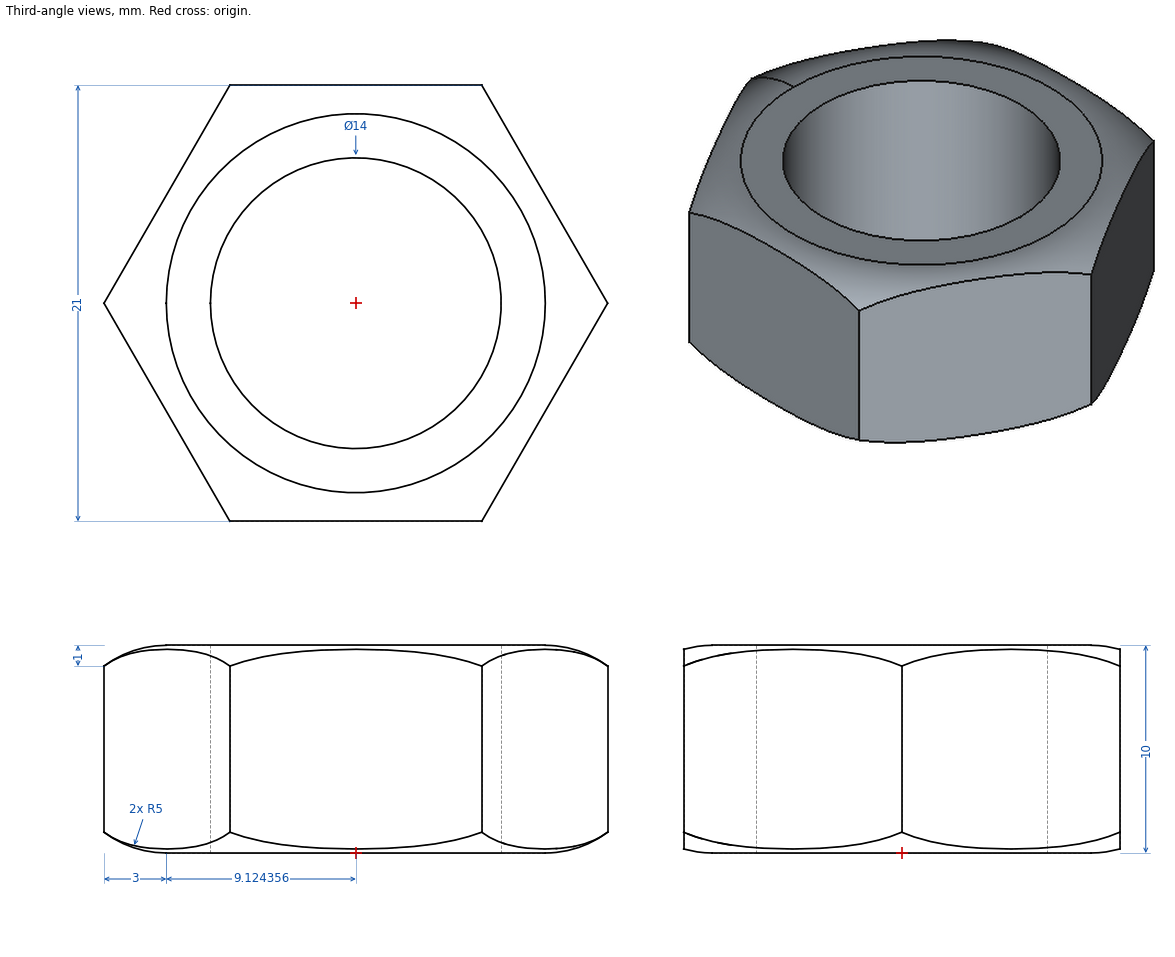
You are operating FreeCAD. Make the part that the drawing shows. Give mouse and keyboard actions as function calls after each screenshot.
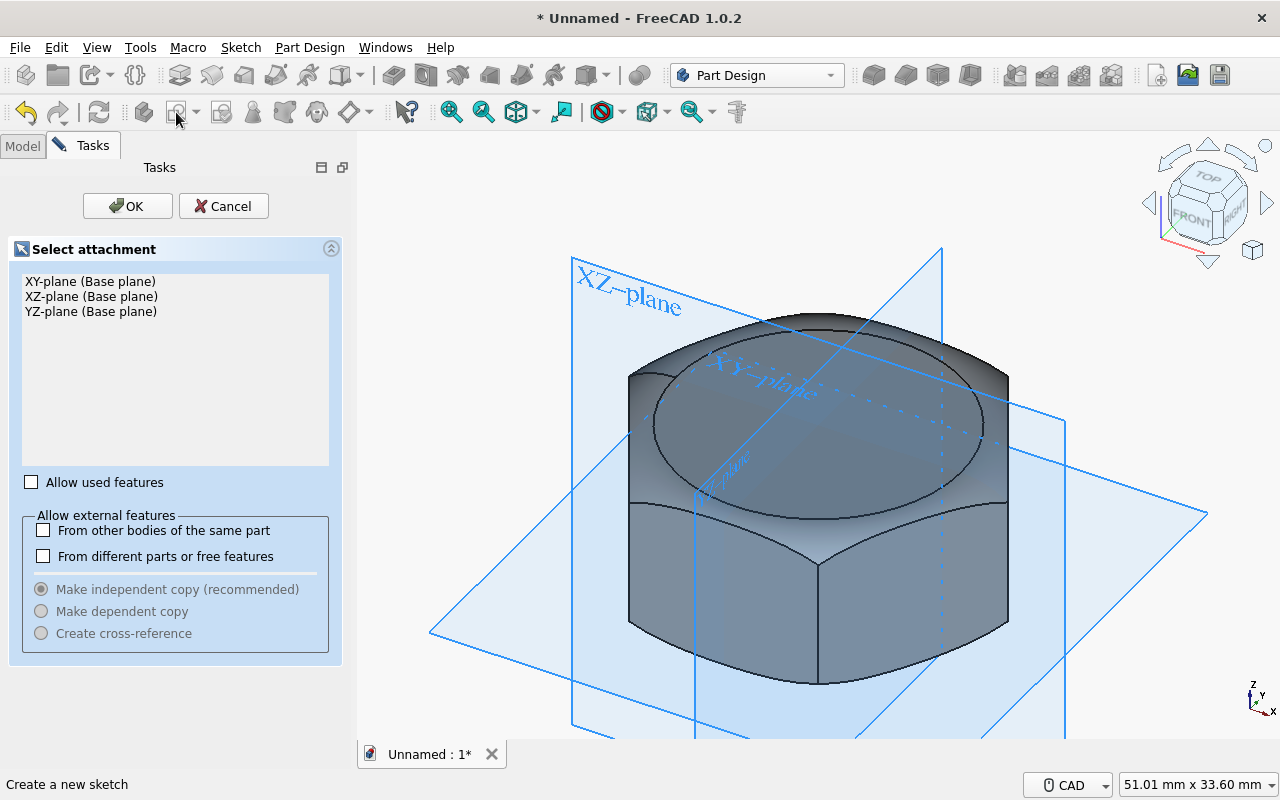
click(82, 282)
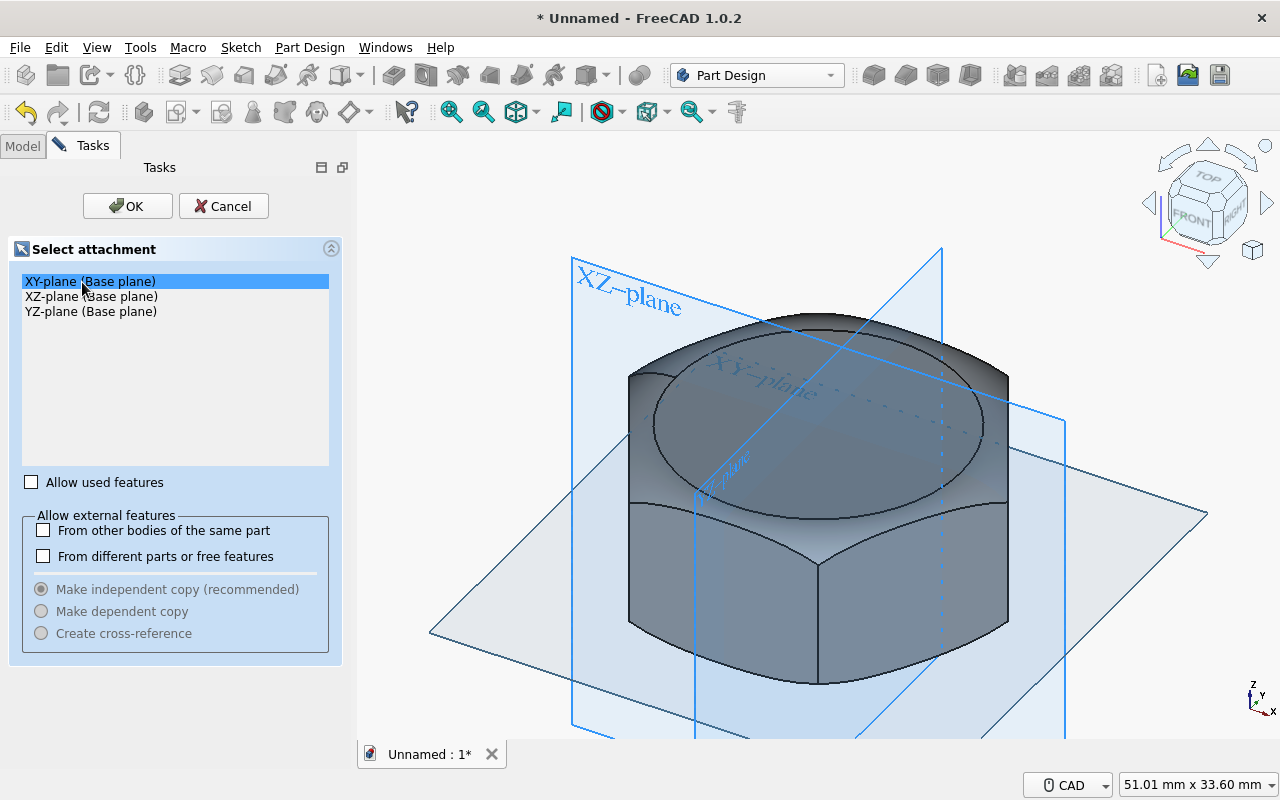
click(128, 206)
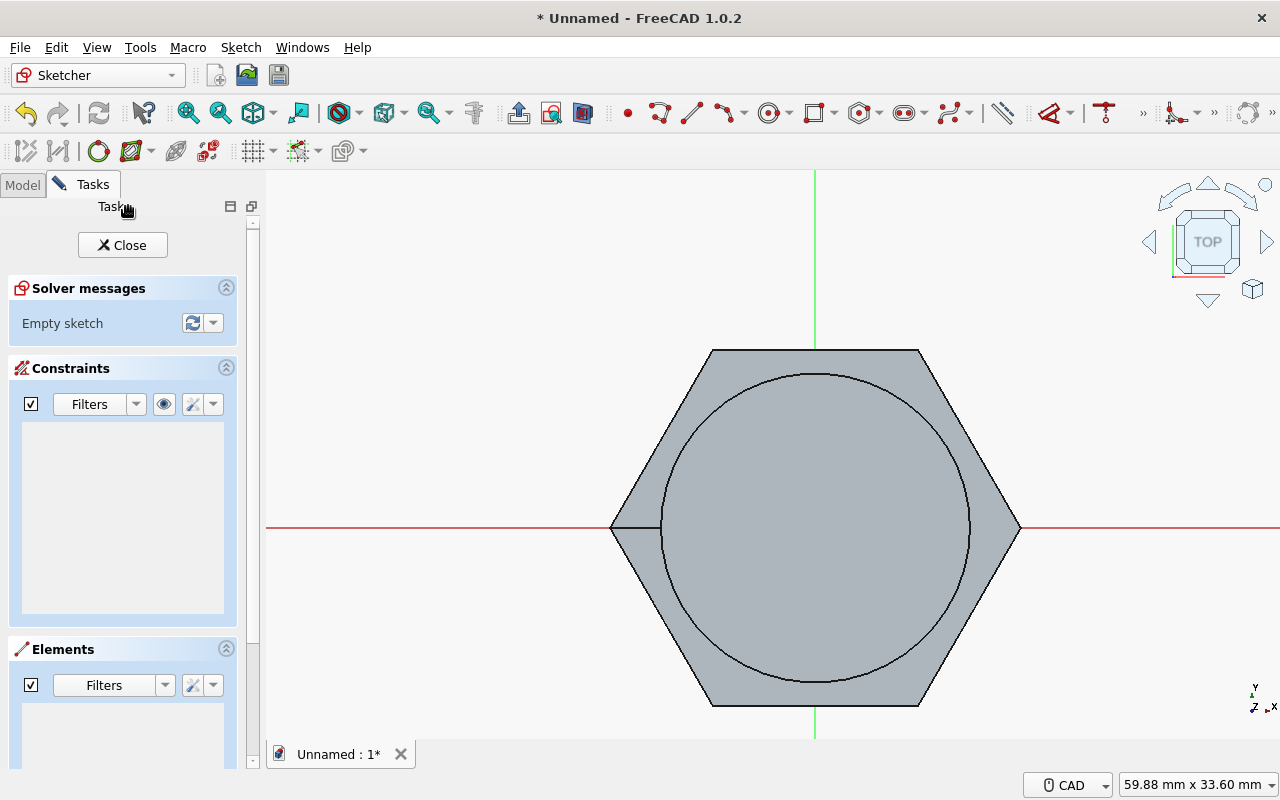
key(q)
key(s)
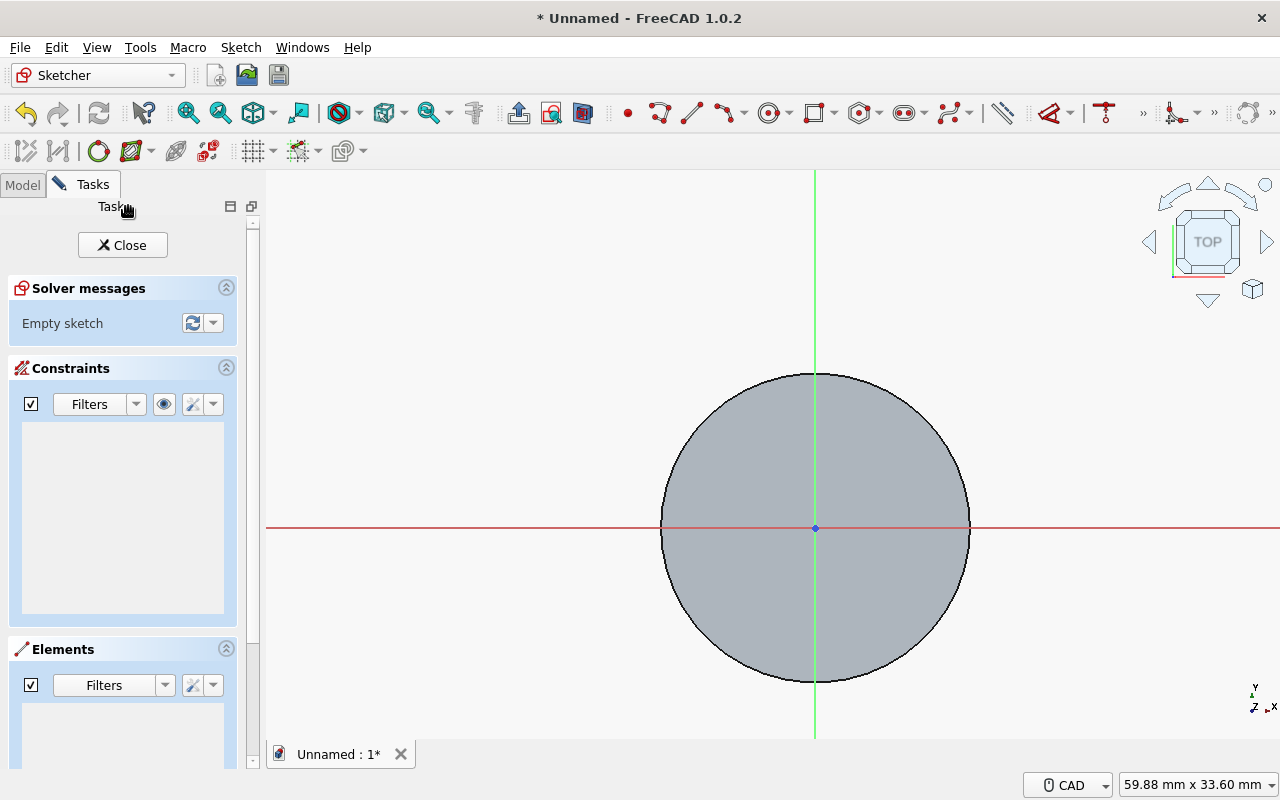
scroll(1041, 678, up, 2)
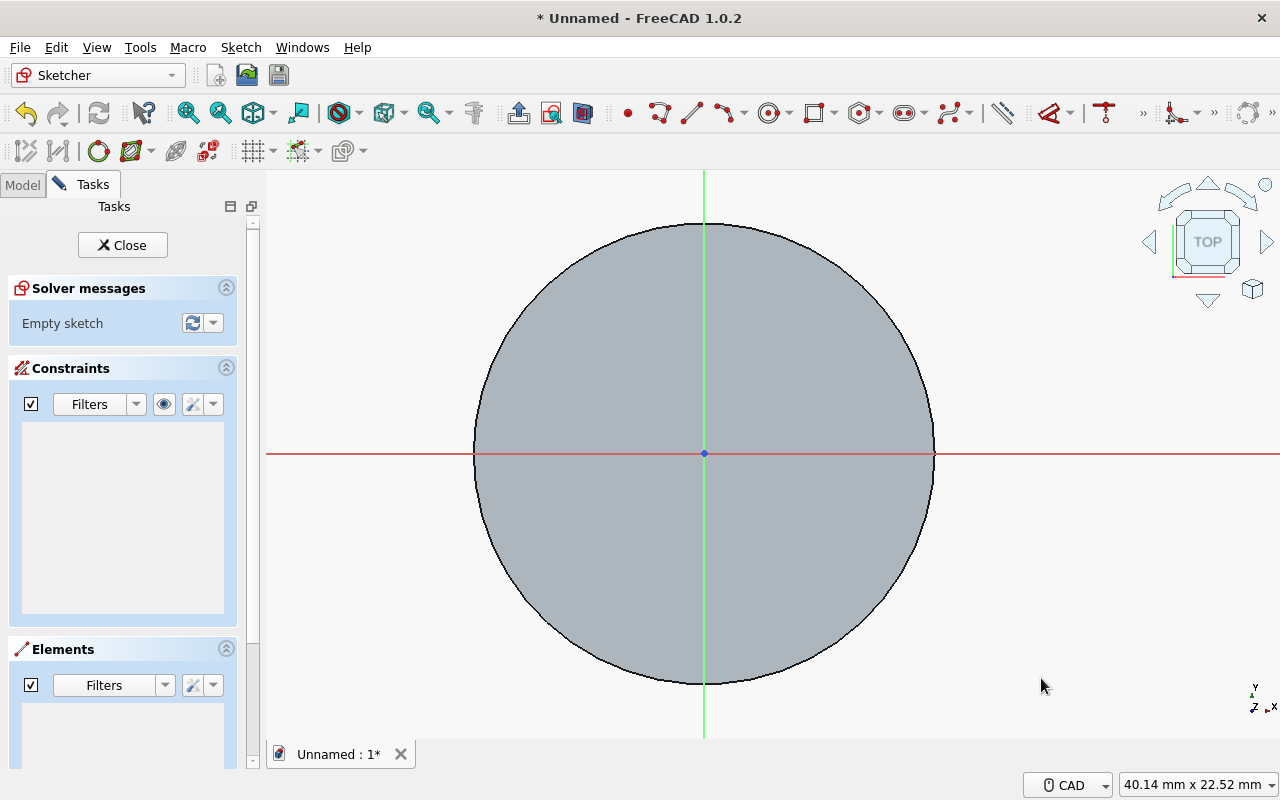
key(g)
key(c)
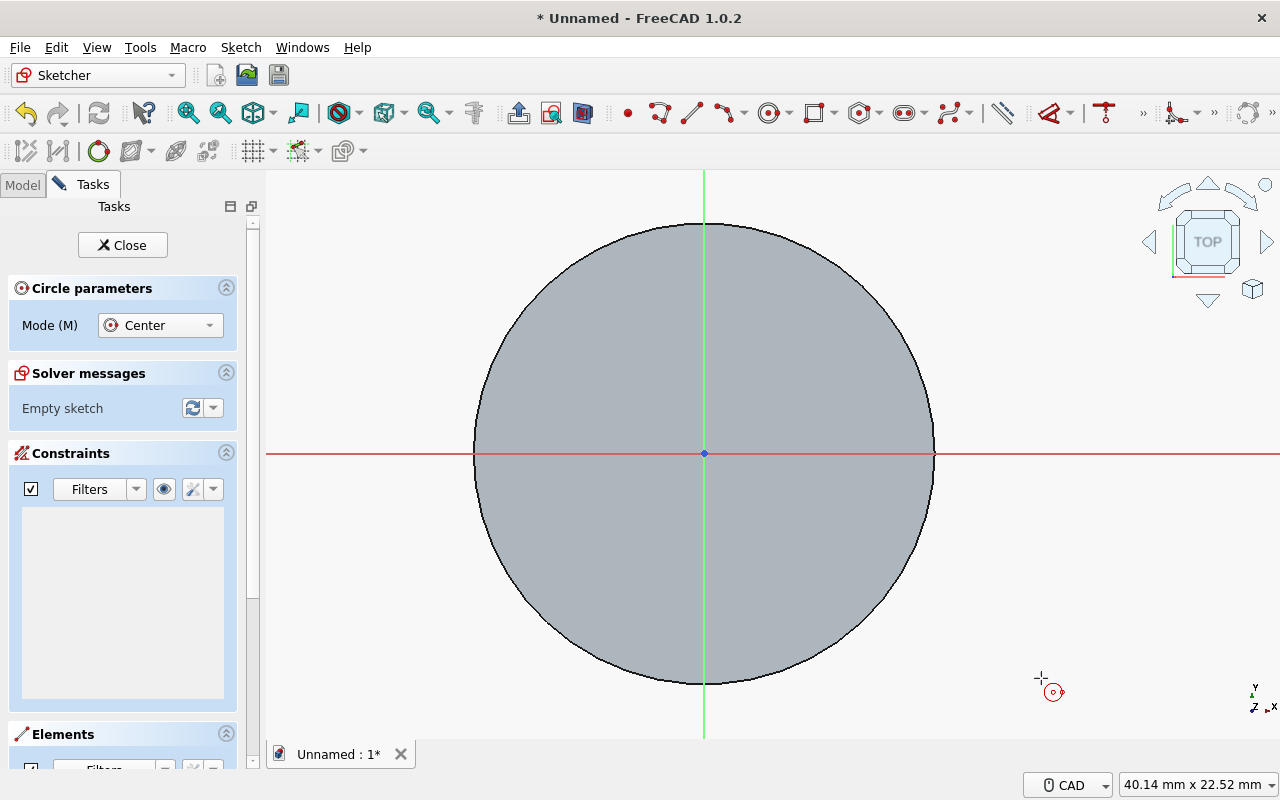
click(704, 454)
move(829, 329)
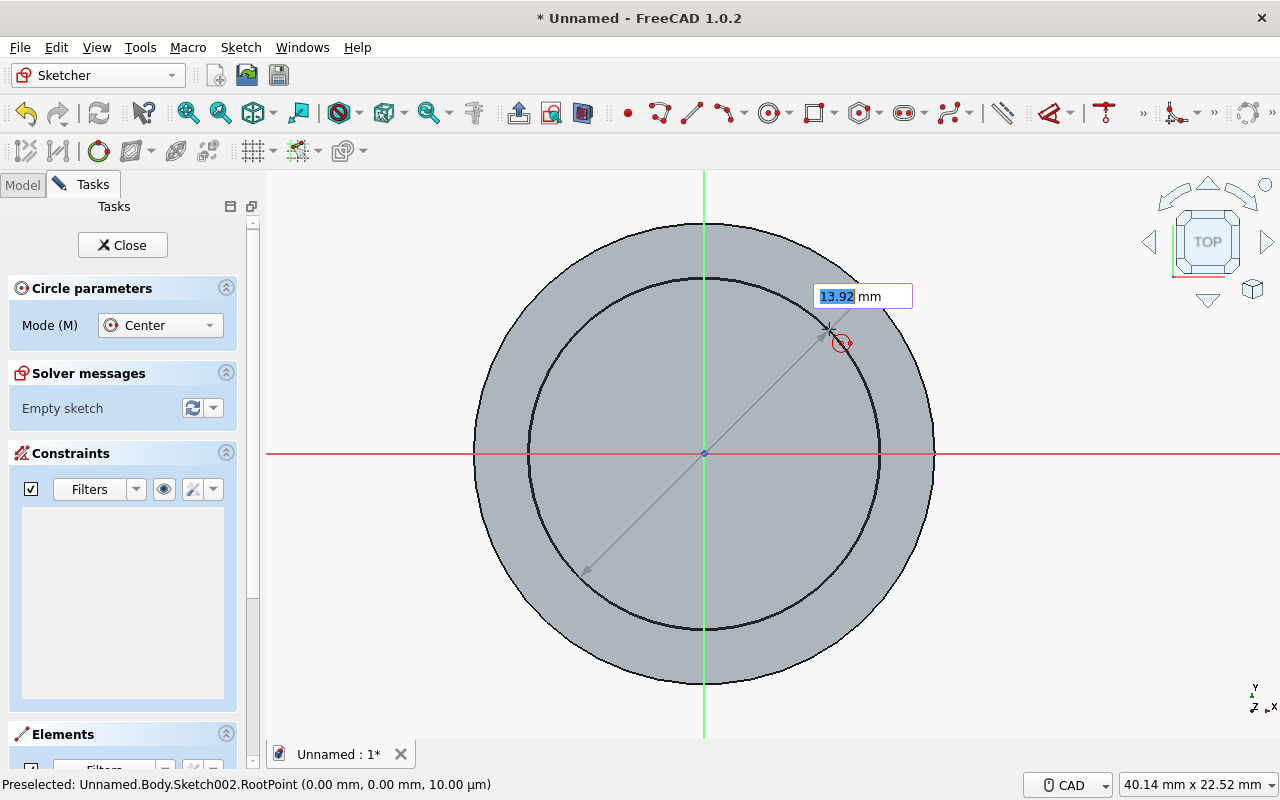
text(14)
key(Return)
key(Escape)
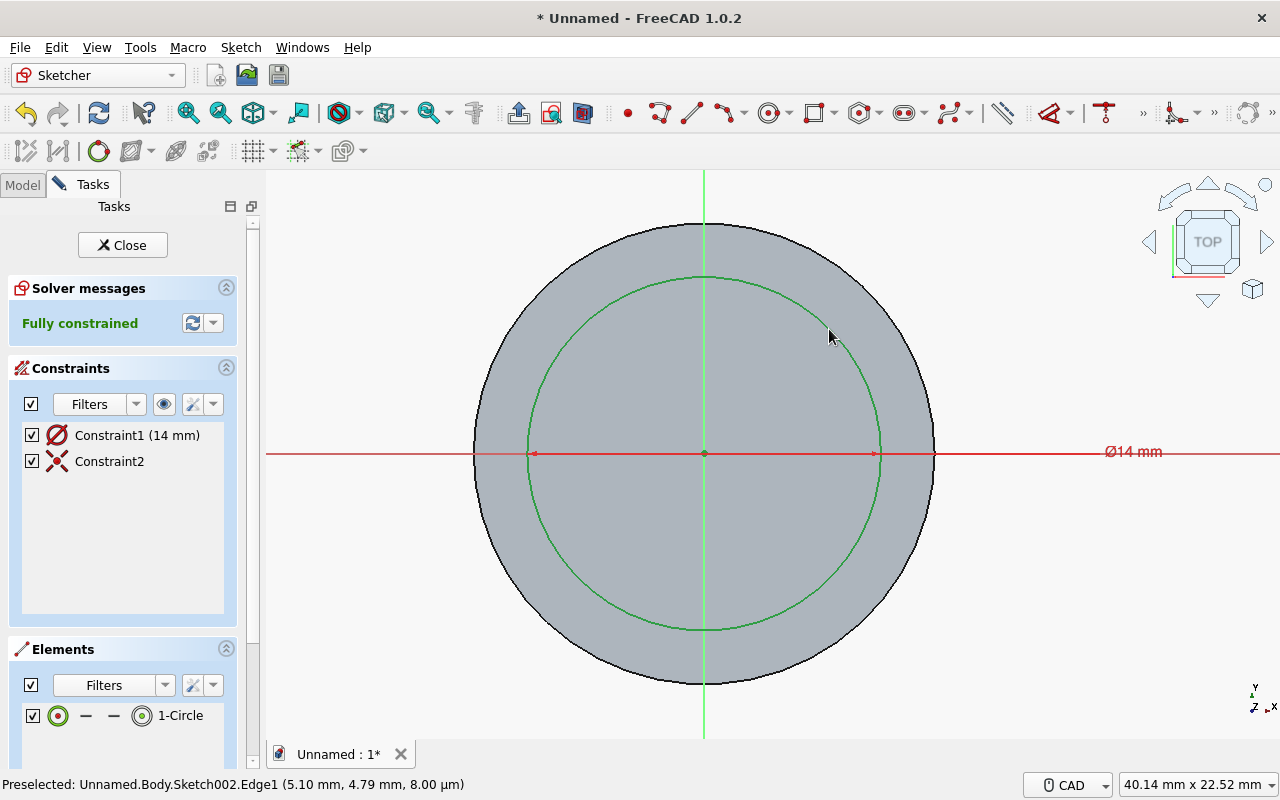
click(123, 245)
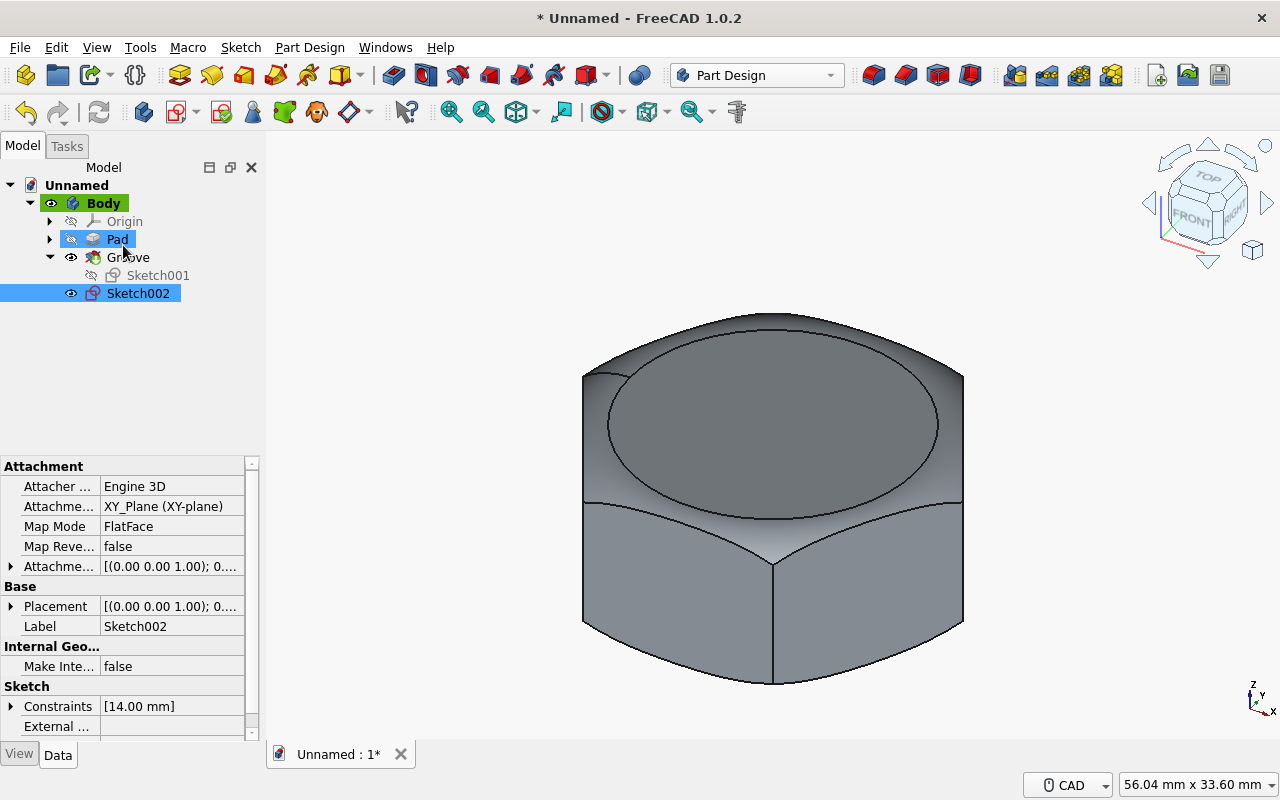
click(394, 76)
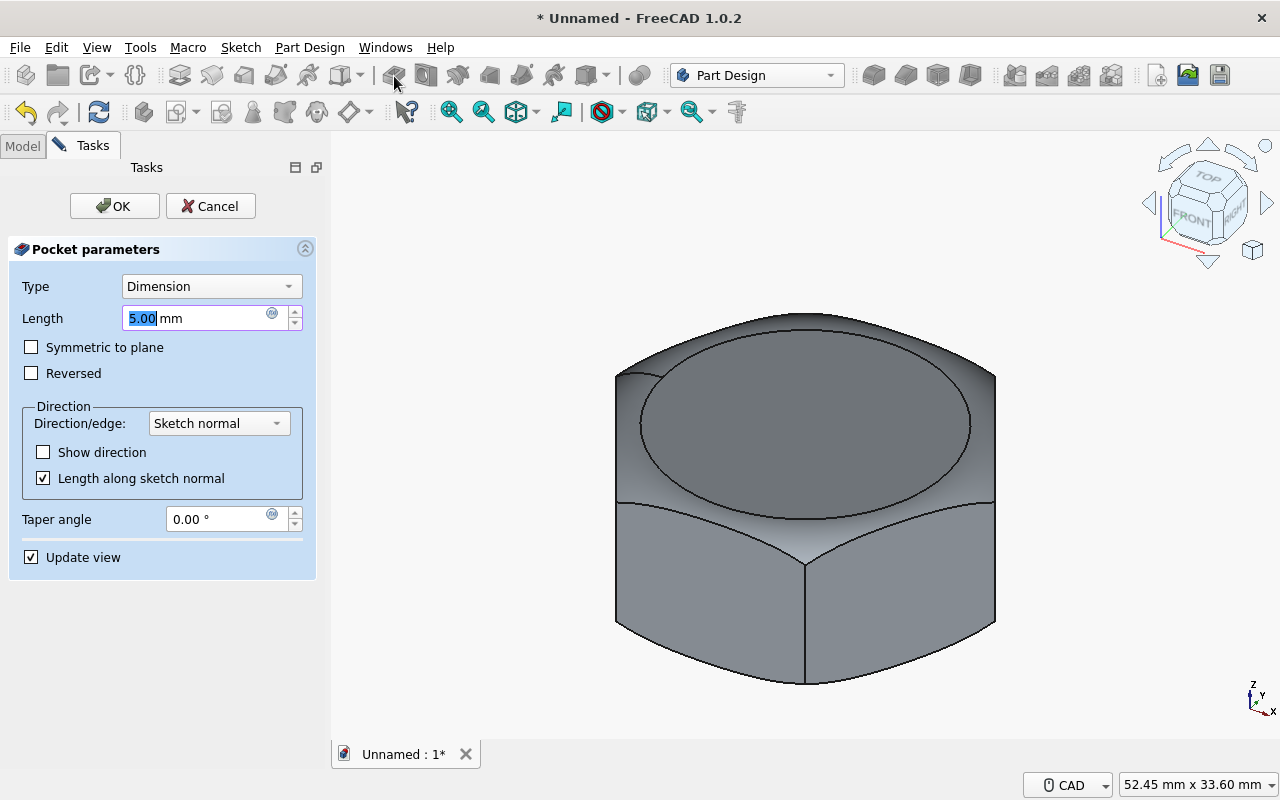
text(10)
key(Tab)